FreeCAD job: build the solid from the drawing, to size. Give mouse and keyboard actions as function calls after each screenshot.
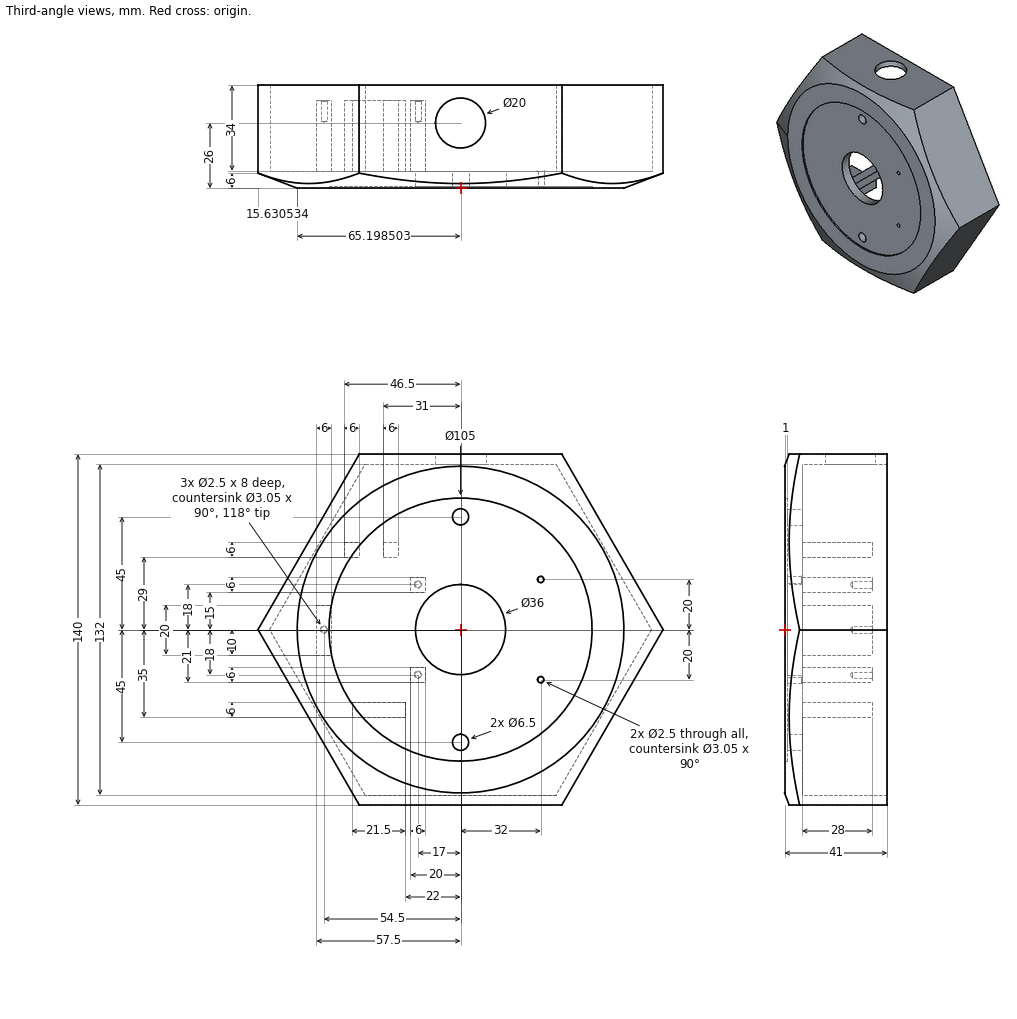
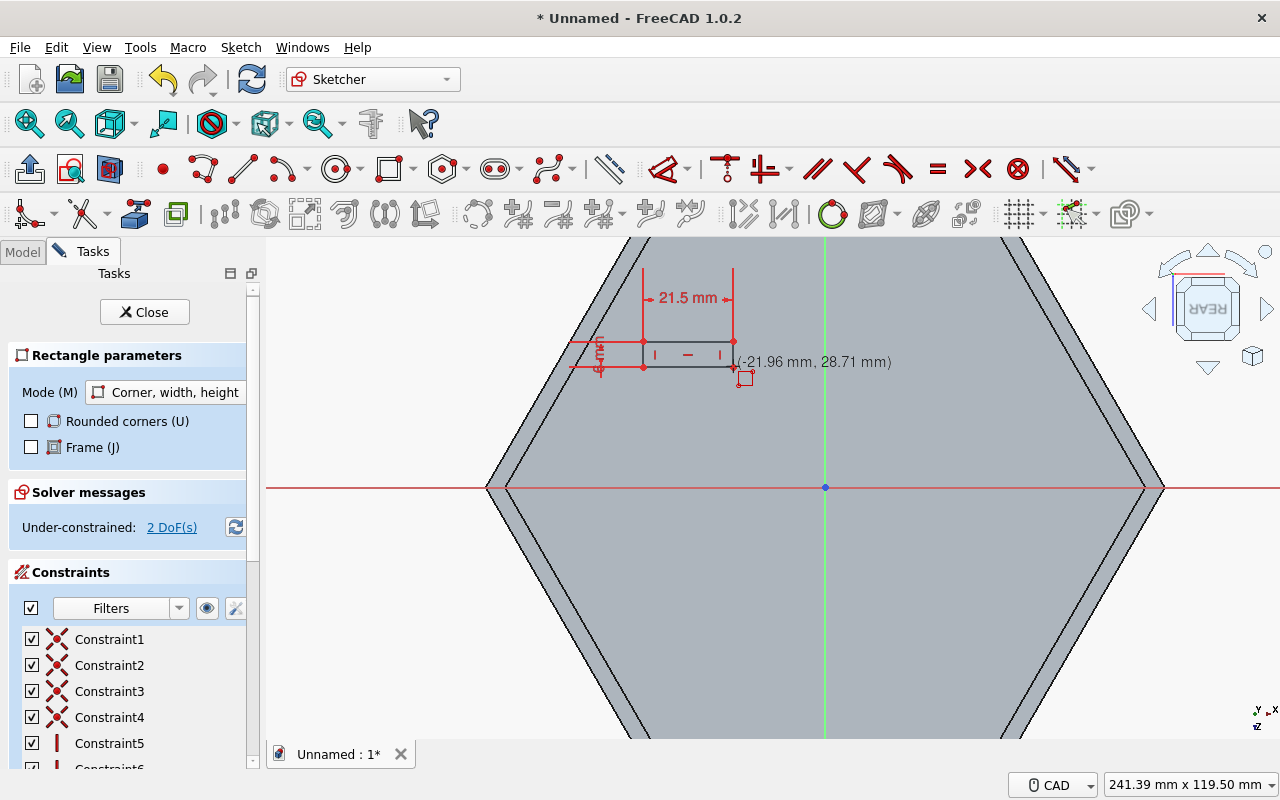
click(584, 446)
move(609, 530)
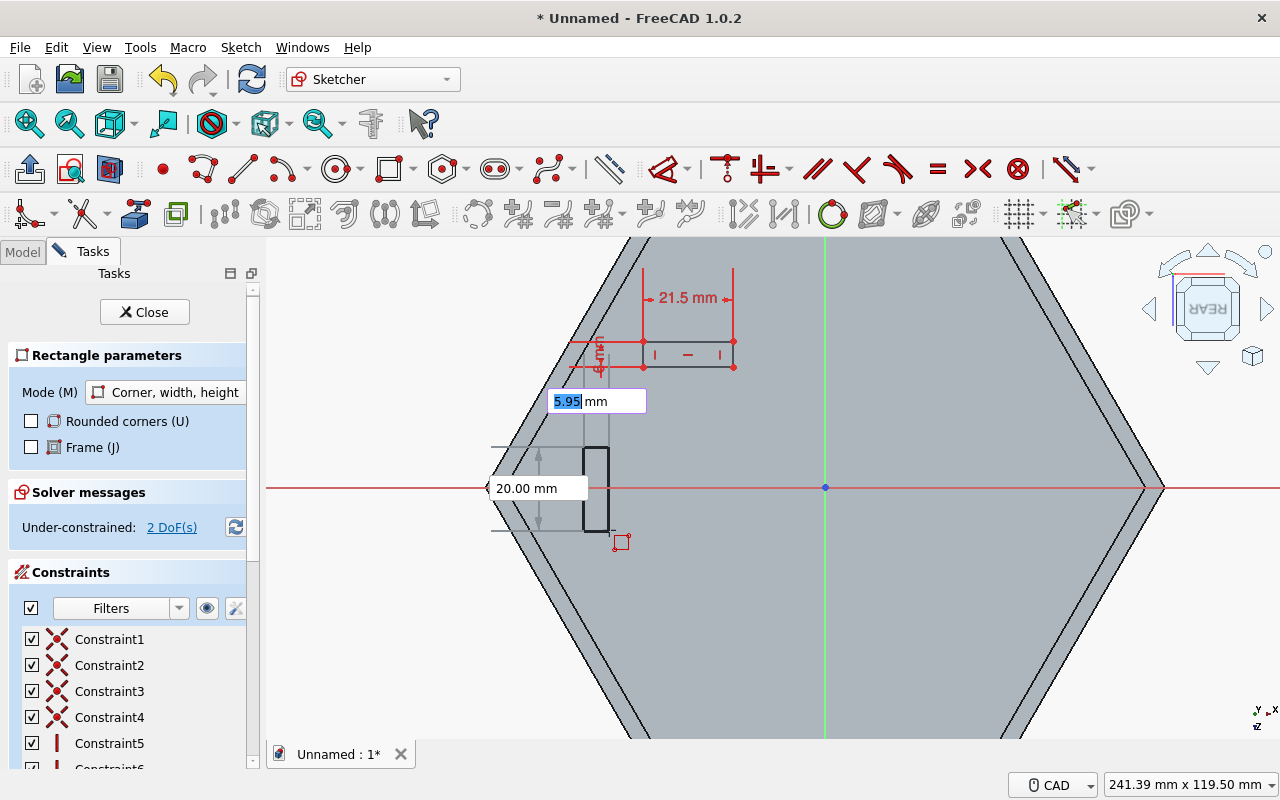
text(6)
key(Tab)
text(20)
key(Return)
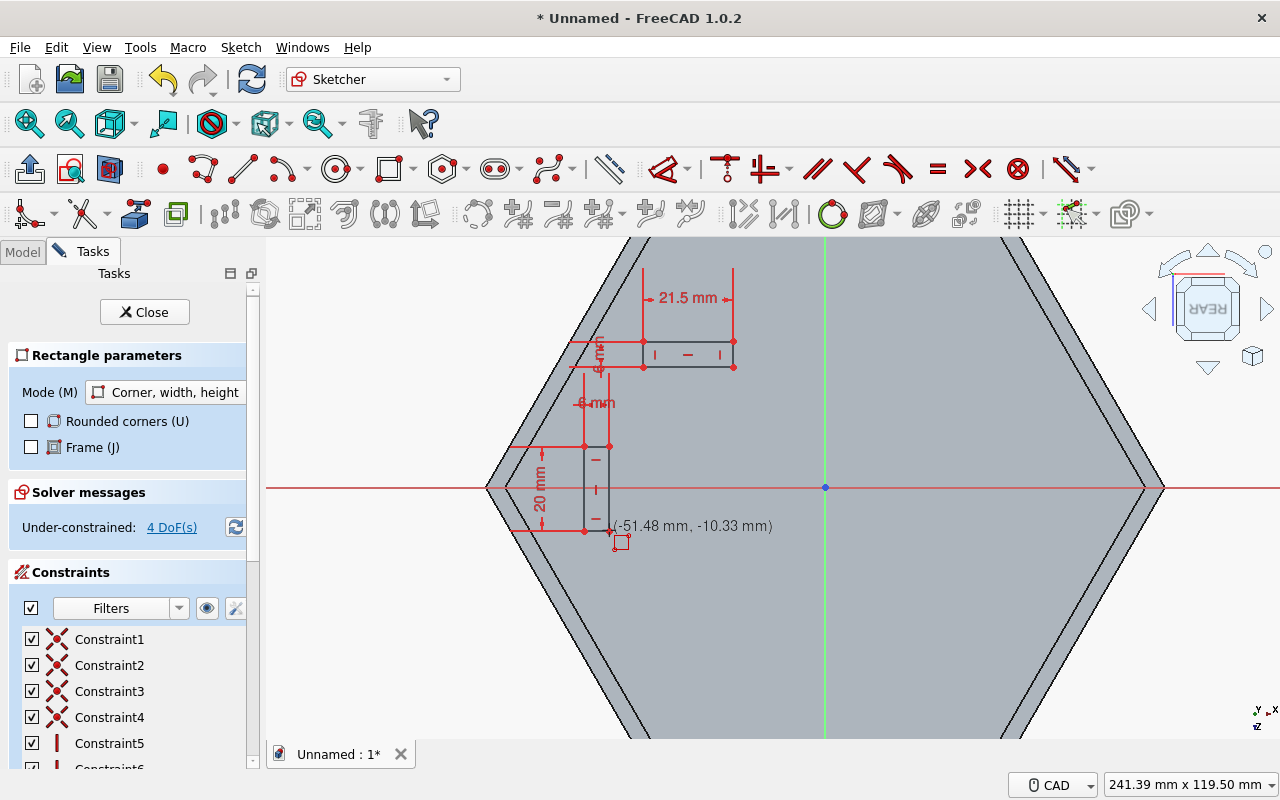
click(630, 609)
move(655, 635)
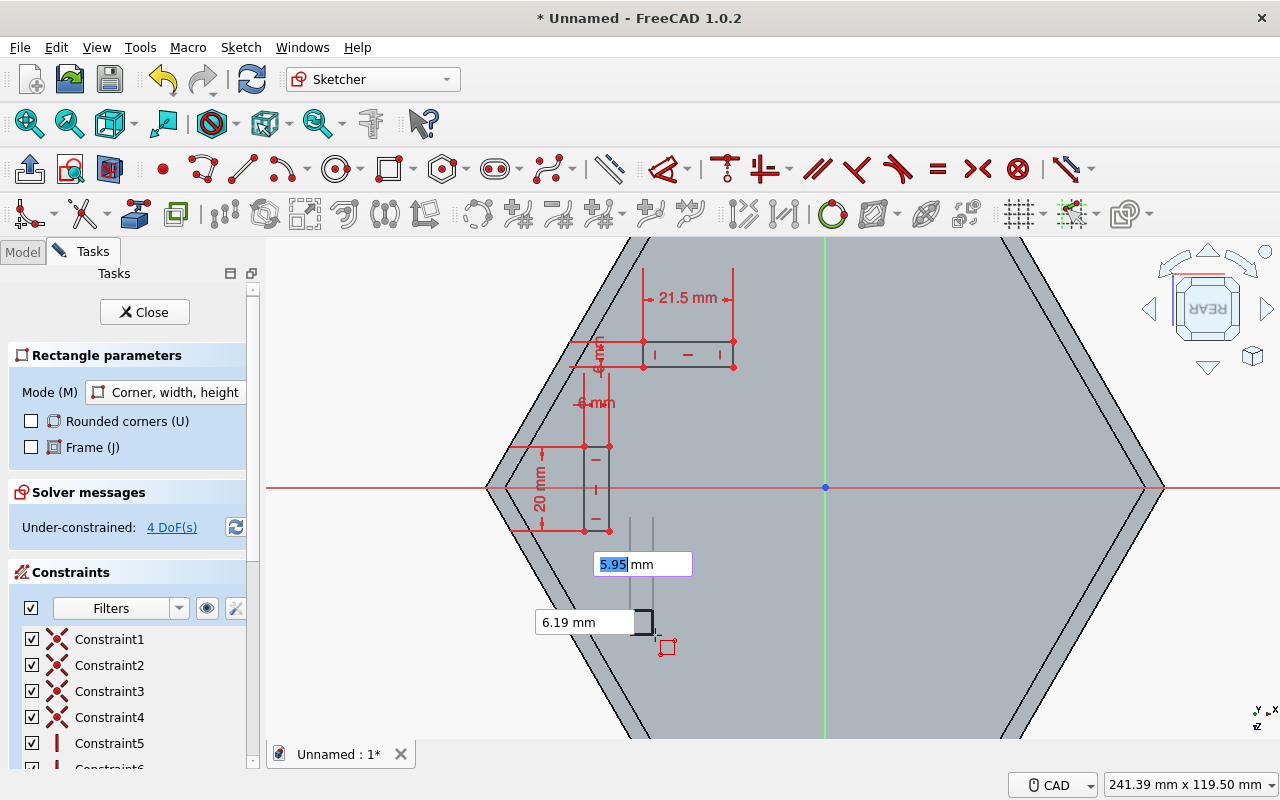
text(6)
key(Tab)
text(6)
key(Return)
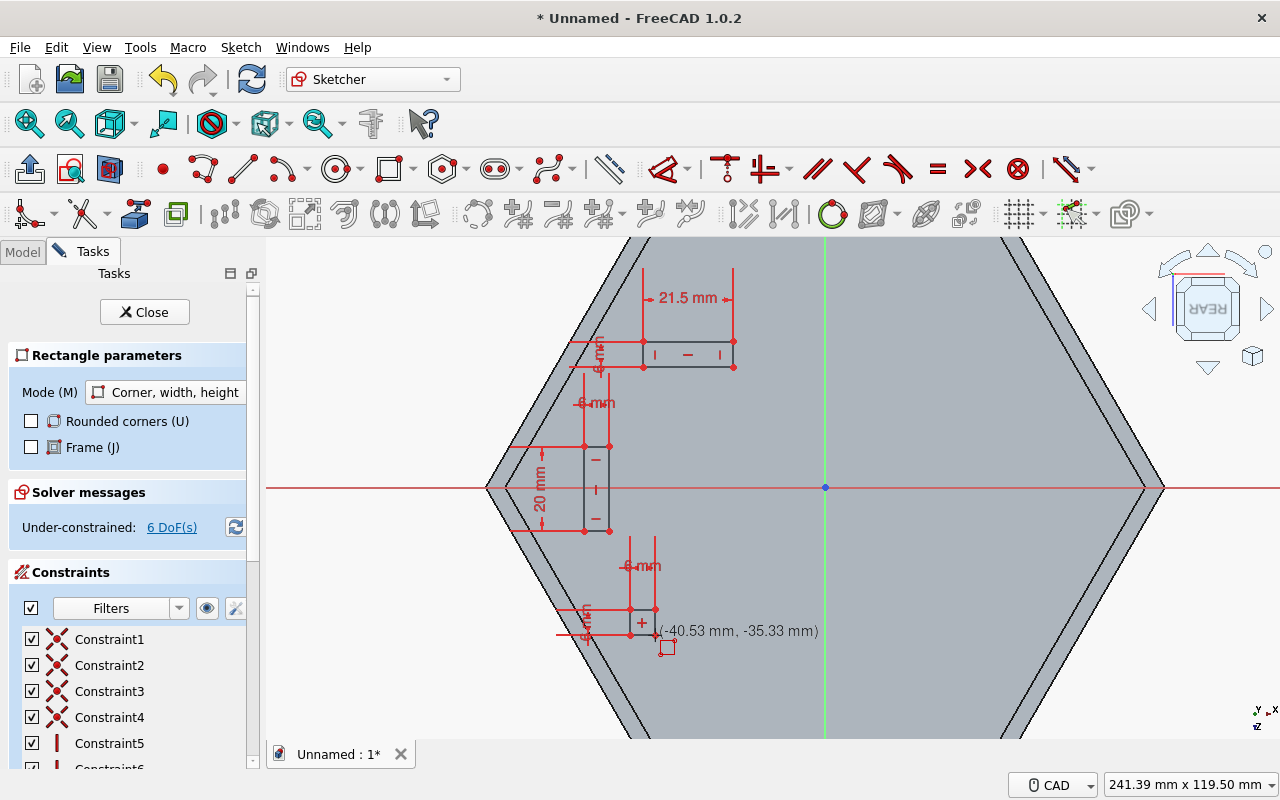
click(695, 609)
move(720, 635)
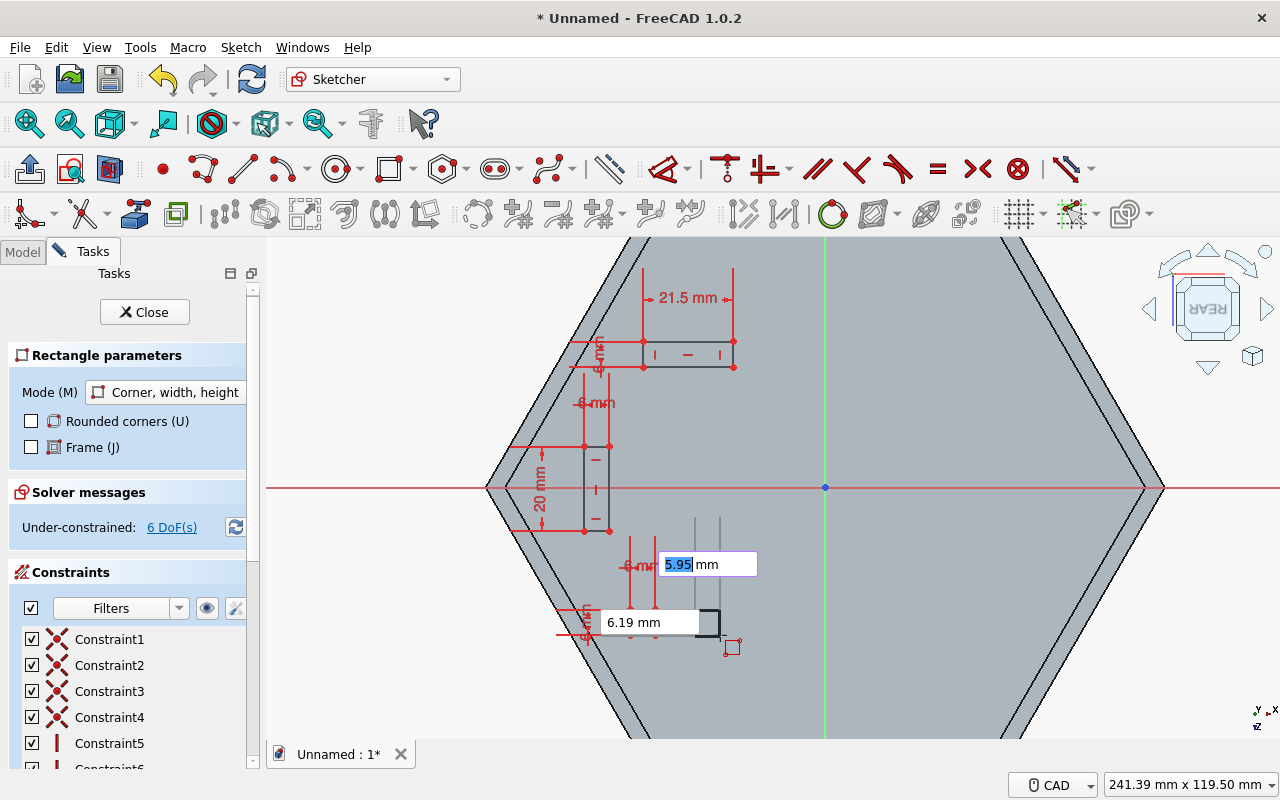
text(6)
key(Tab)
text(6)
key(Return)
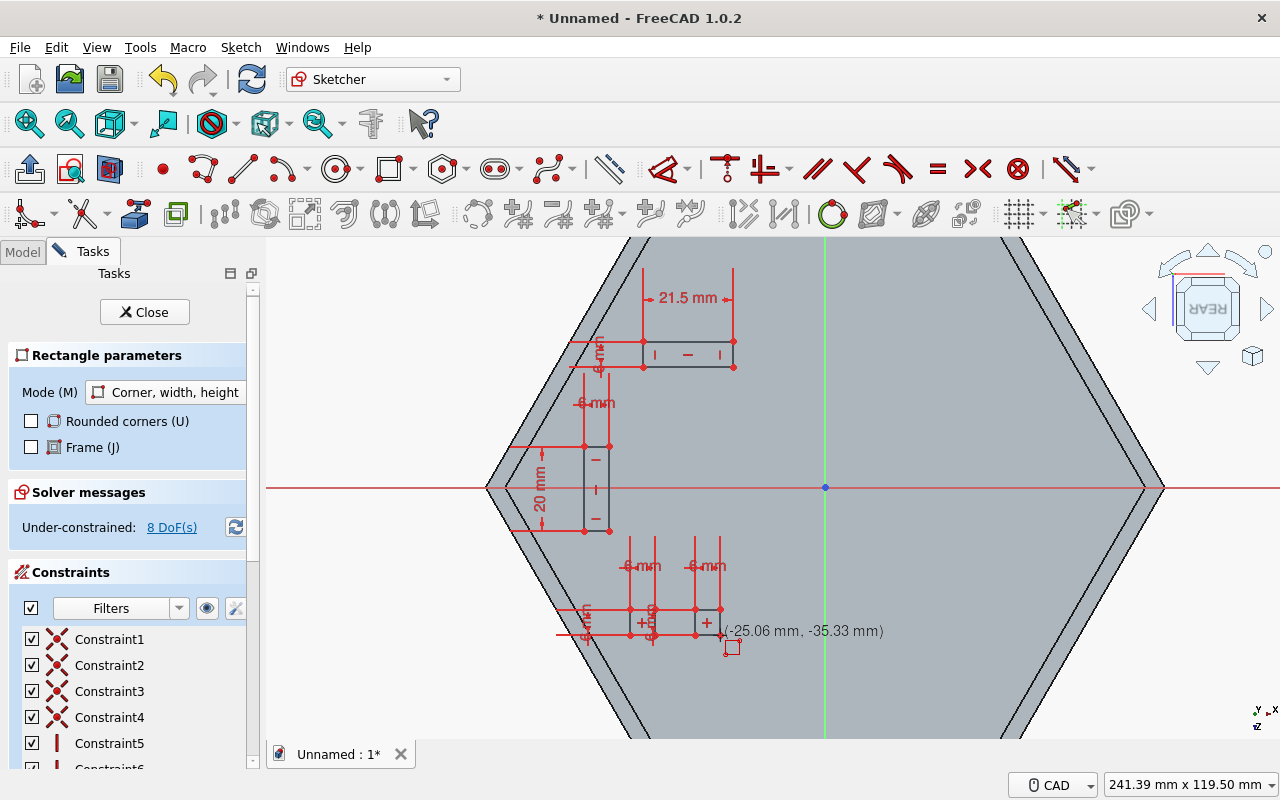
click(741, 399)
move(766, 425)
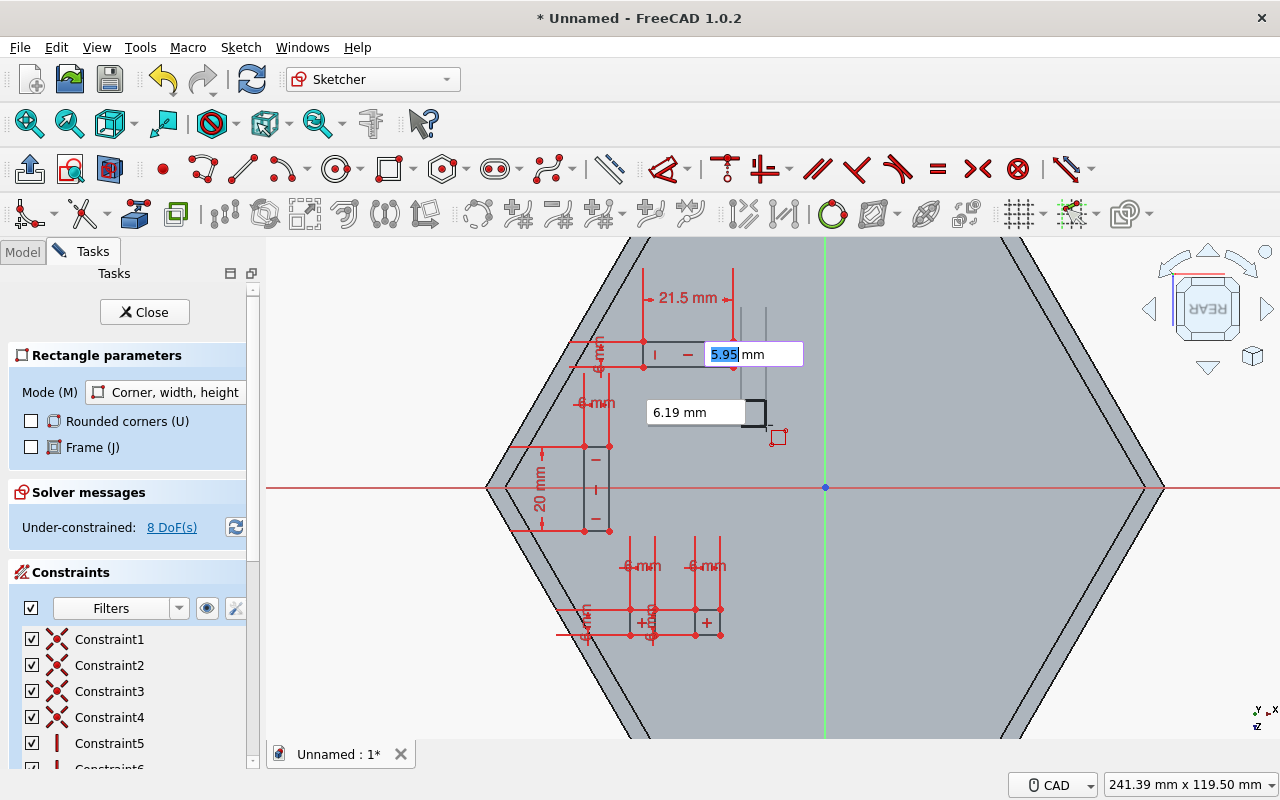
text(6)
key(Tab)
text(6)
key(Return)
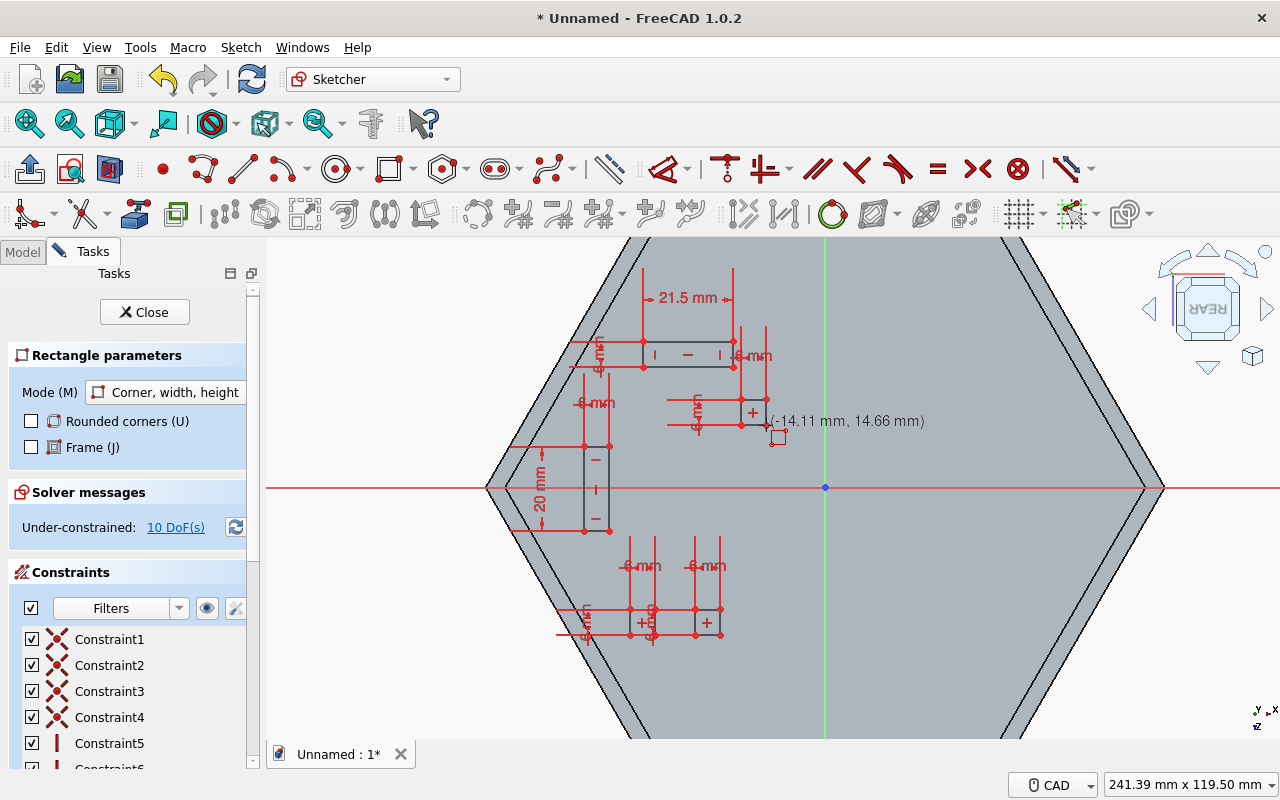
click(741, 551)
move(766, 576)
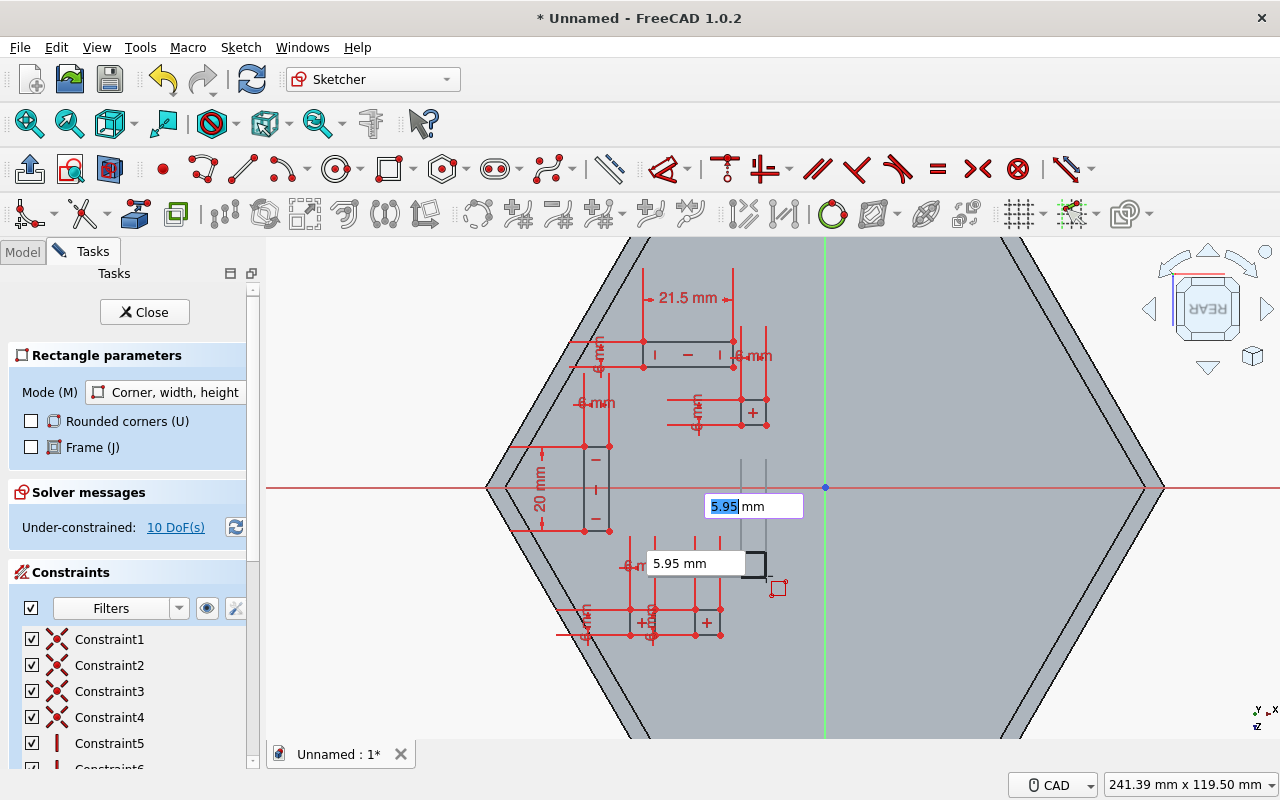
text(6)
key(Tab)
text(6)
key(Return)
key(Escape)